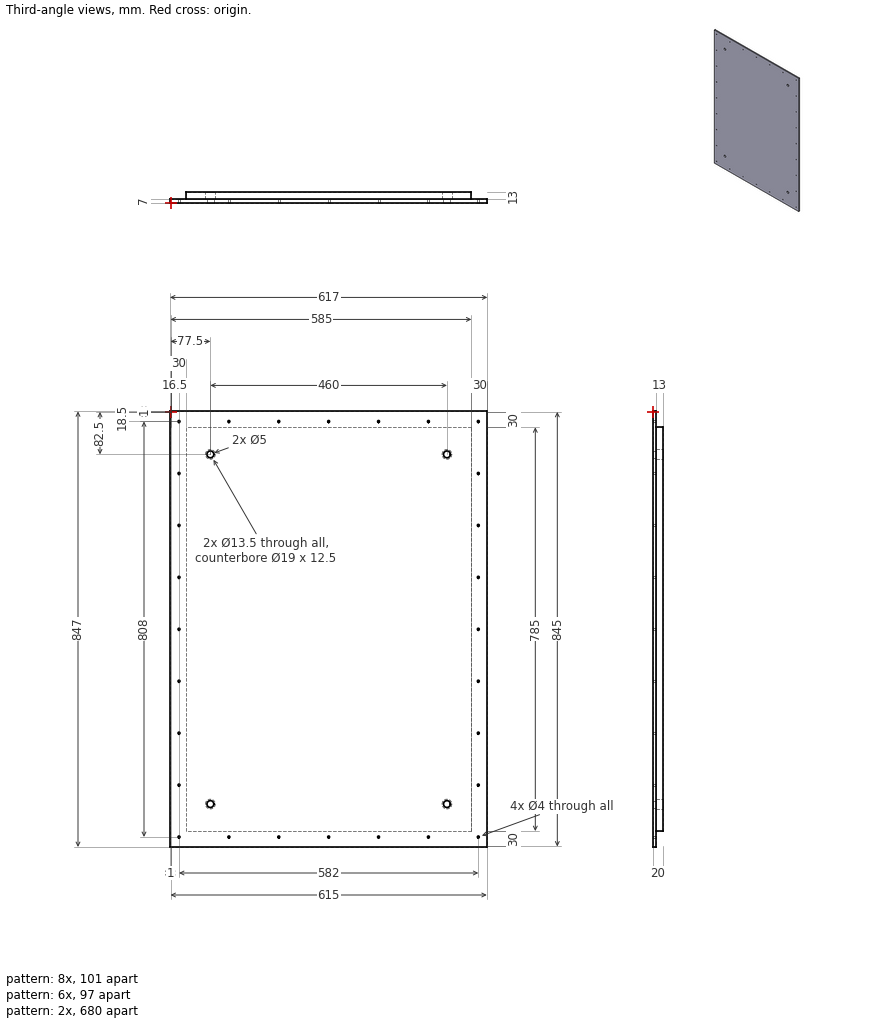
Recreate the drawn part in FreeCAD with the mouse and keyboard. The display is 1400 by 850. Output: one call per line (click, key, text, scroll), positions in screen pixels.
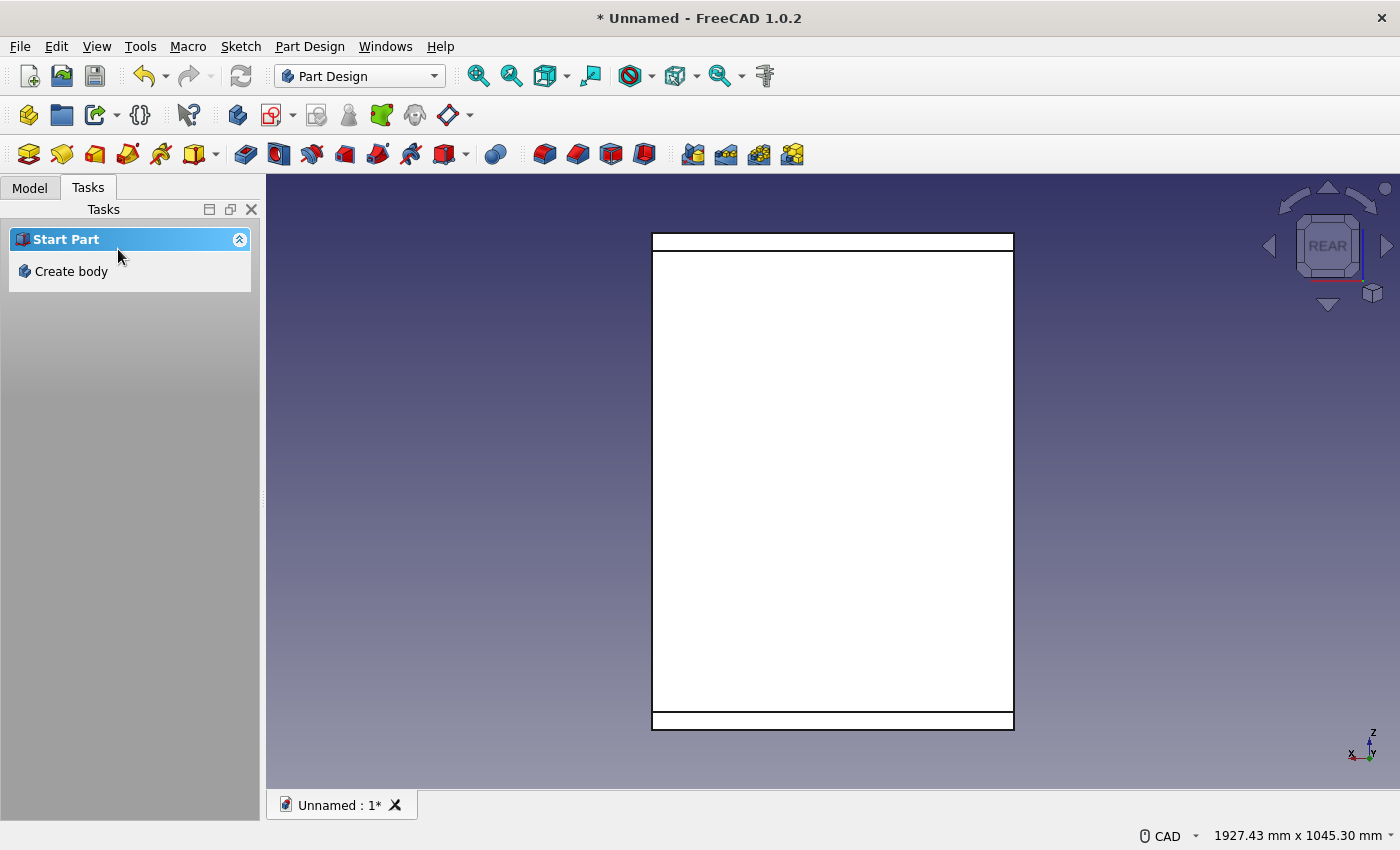
click(833, 480)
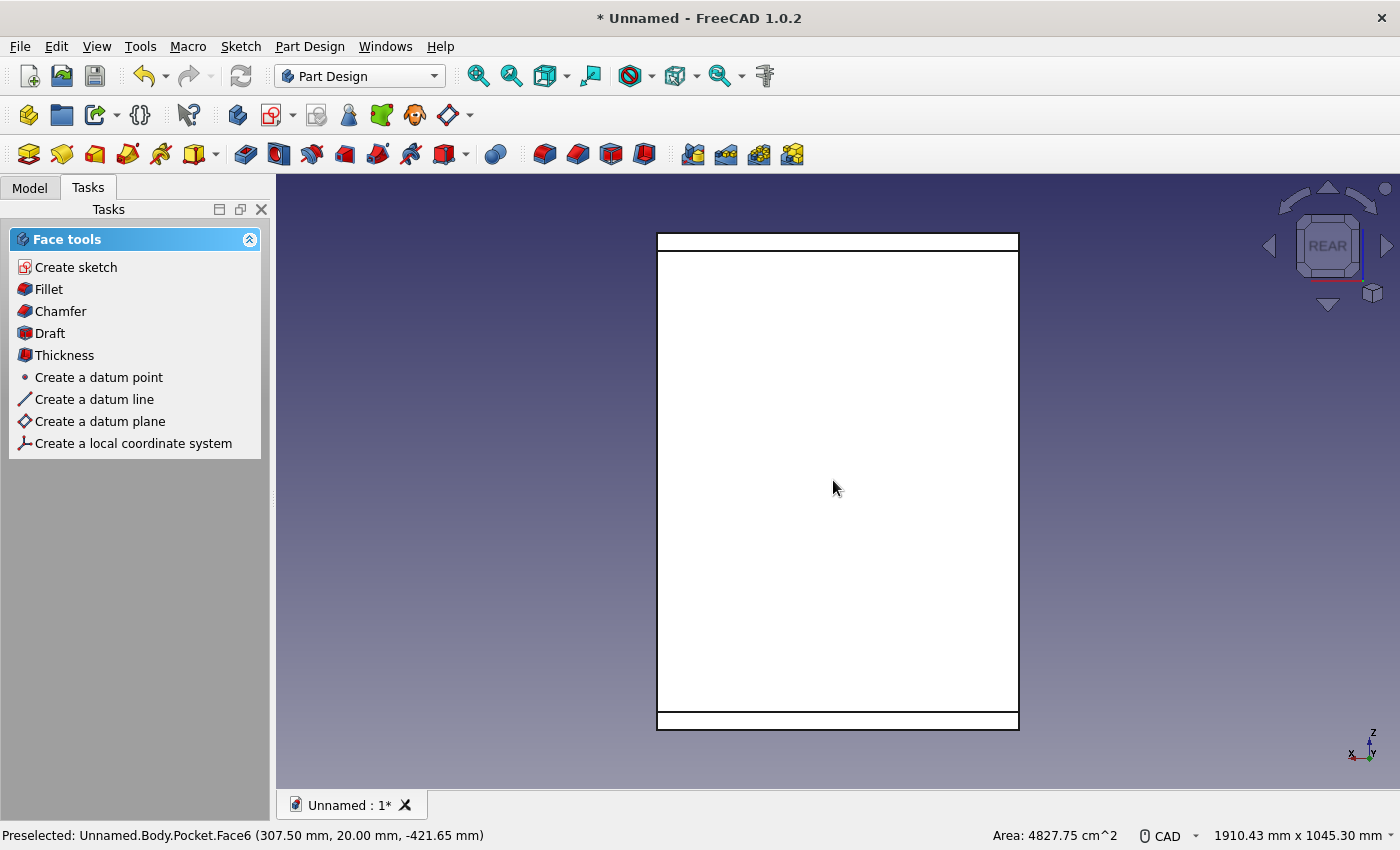
click(270, 116)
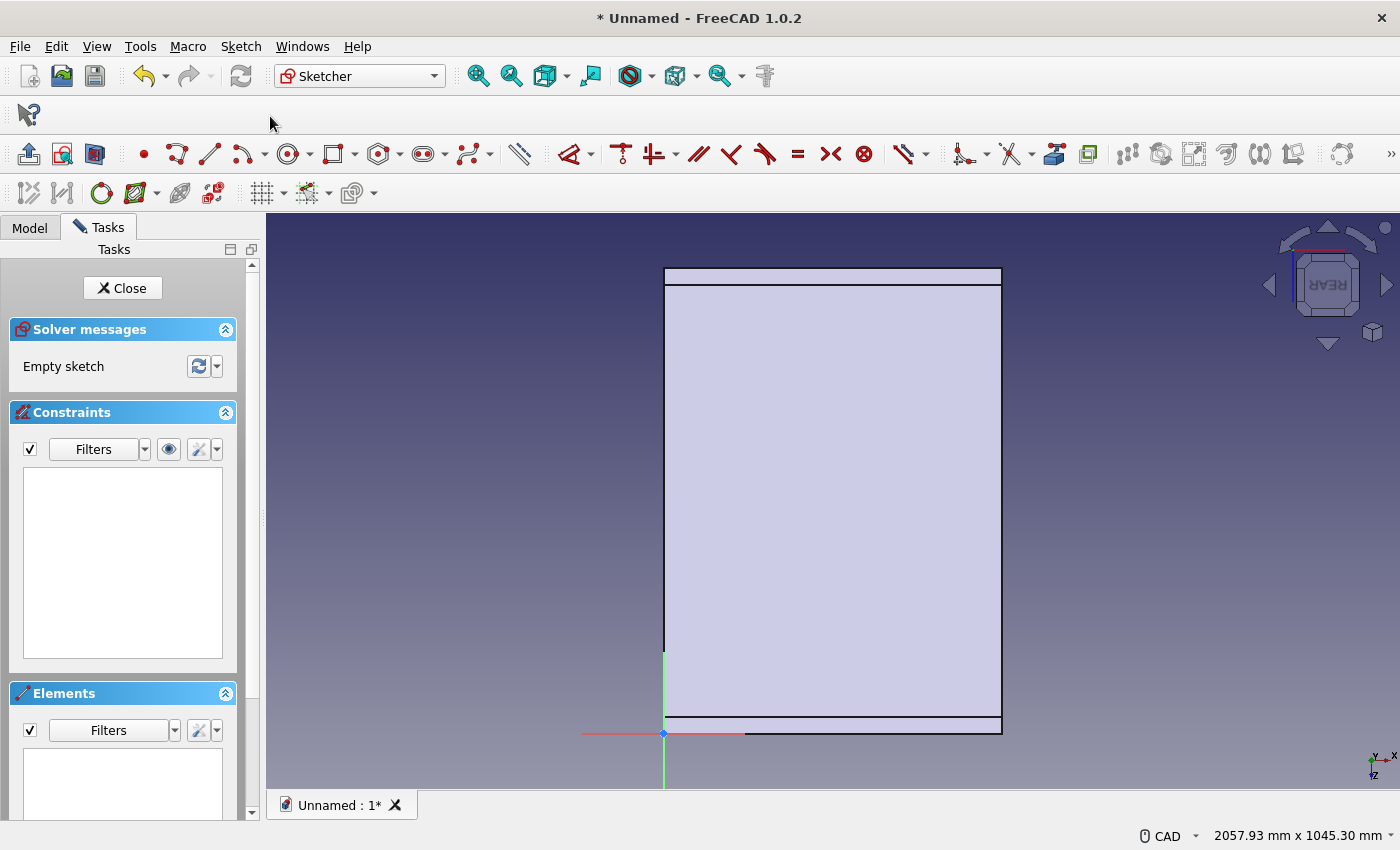
key(g)
key(r)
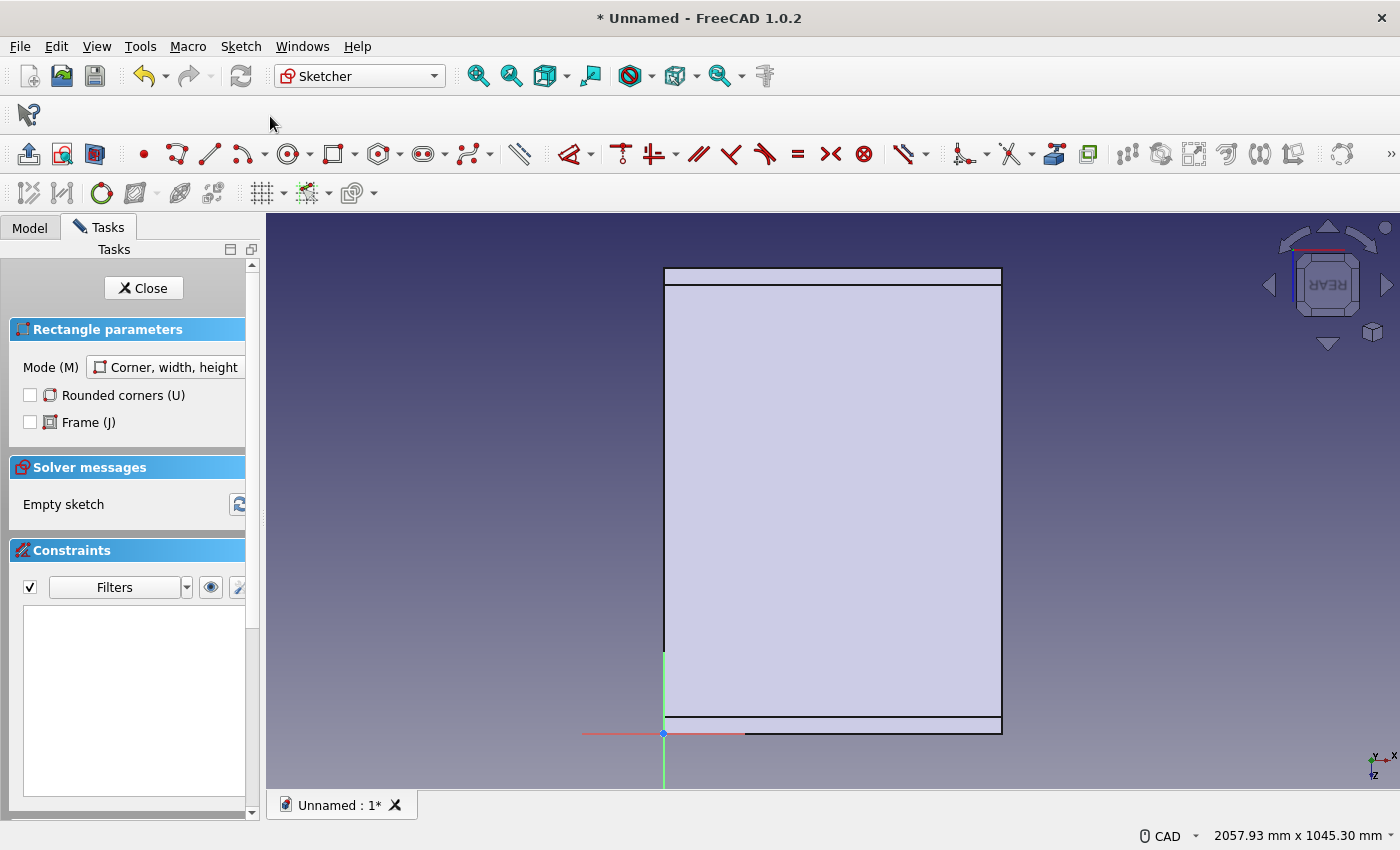
click(986, 285)
move(1002, 717)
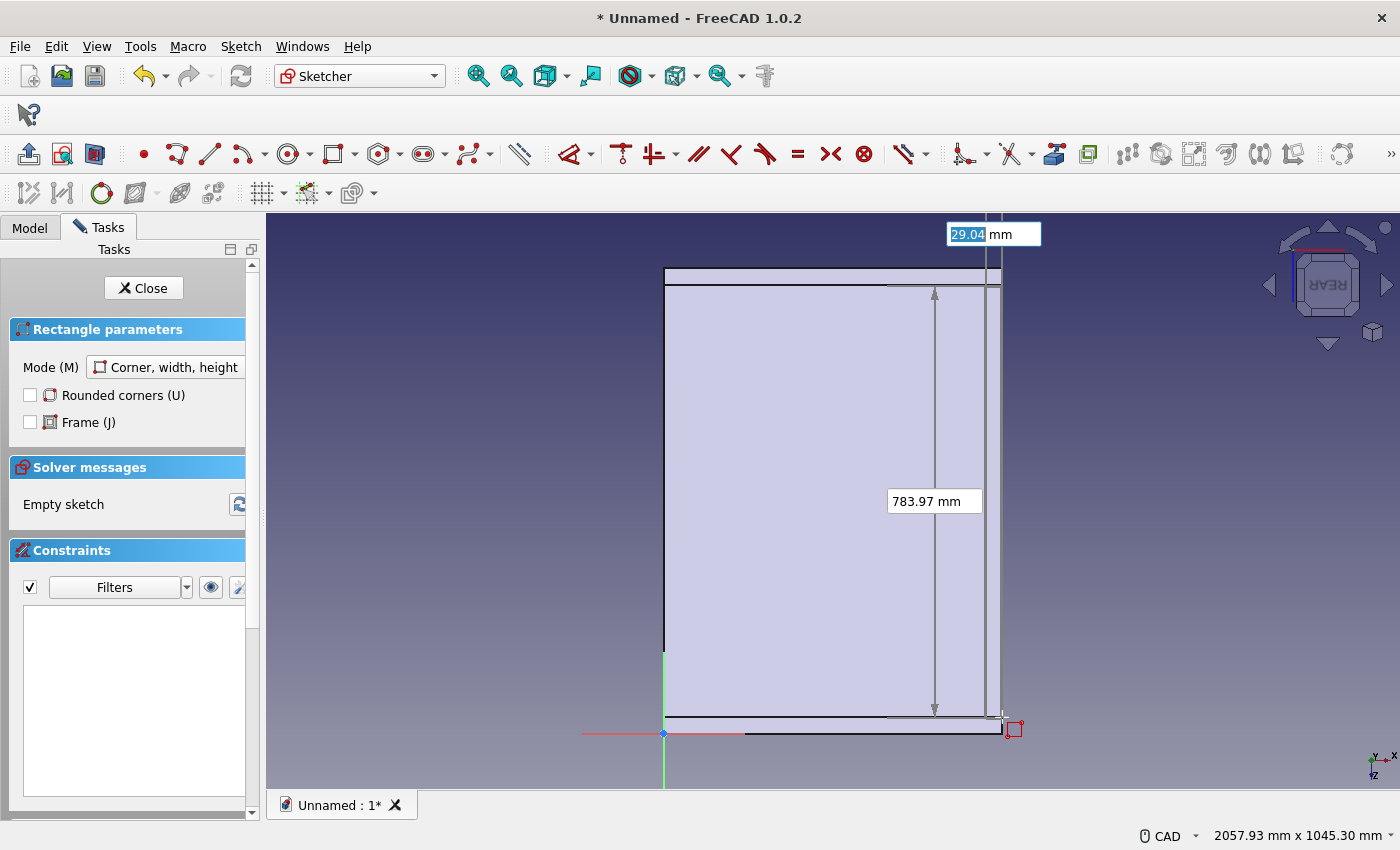
text(30)
key(Tab)
text(785)
key(Return)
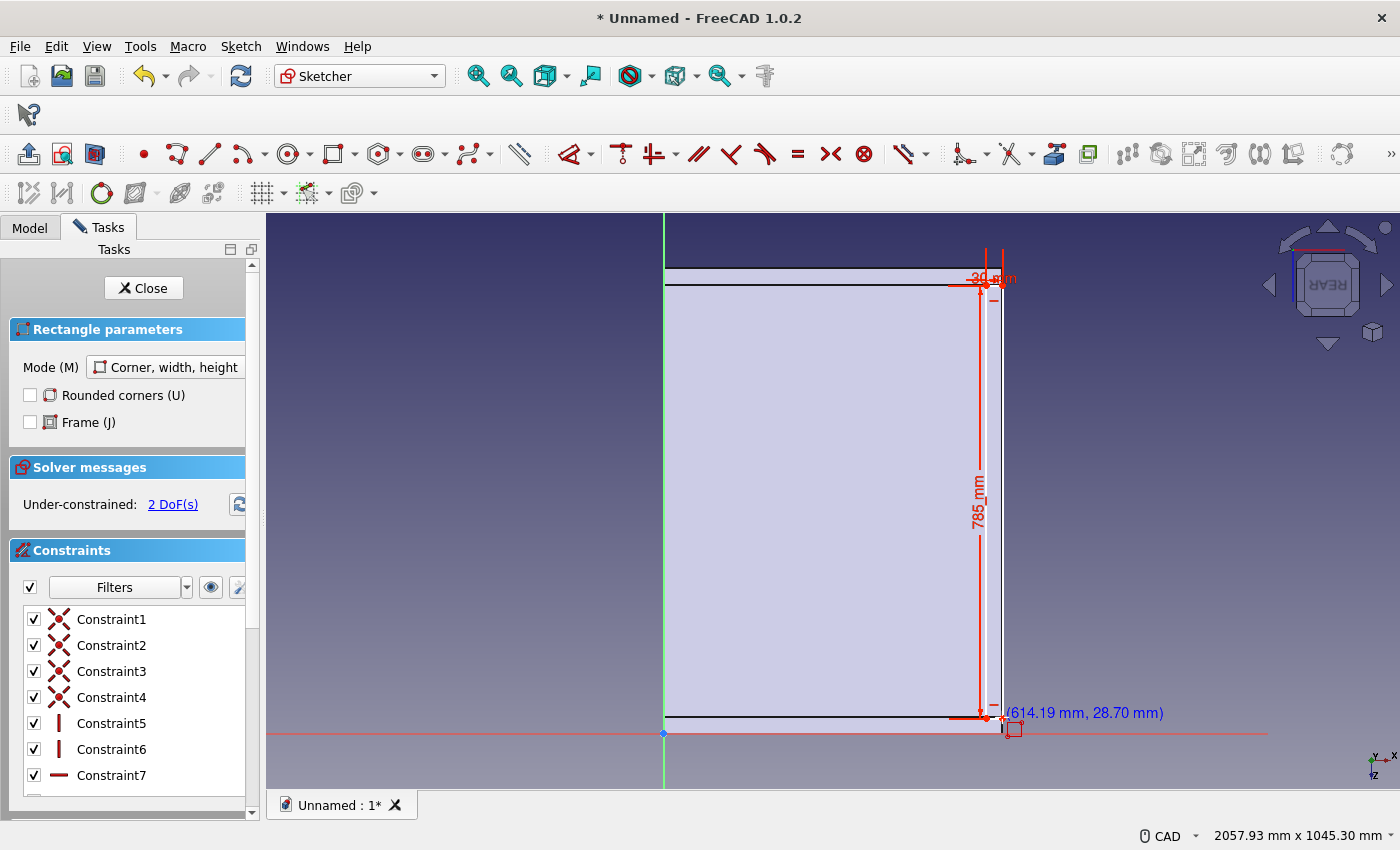
click(664, 285)
move(680, 717)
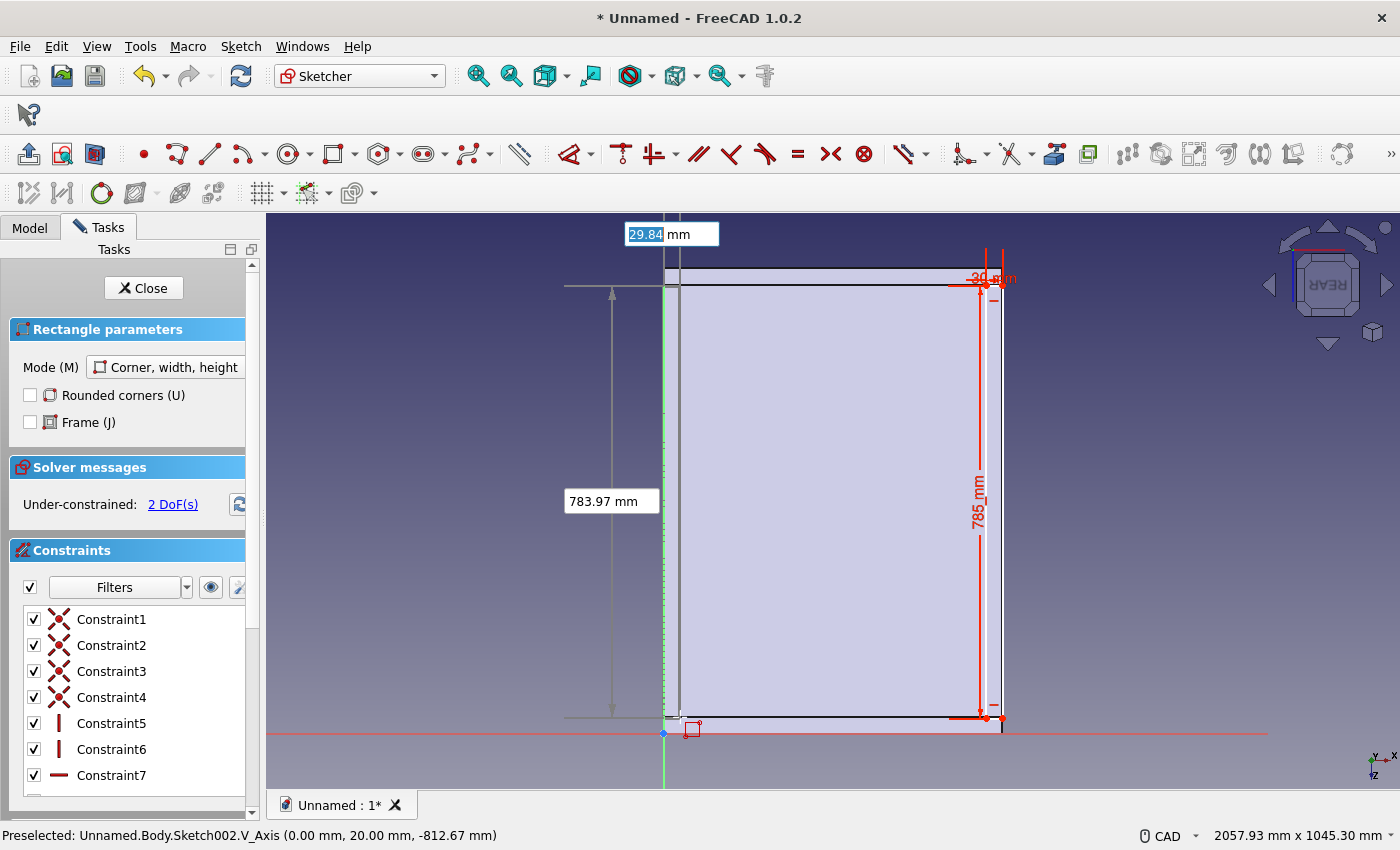
text(30)
key(Tab)
text(785)
key(Return)
key(Escape)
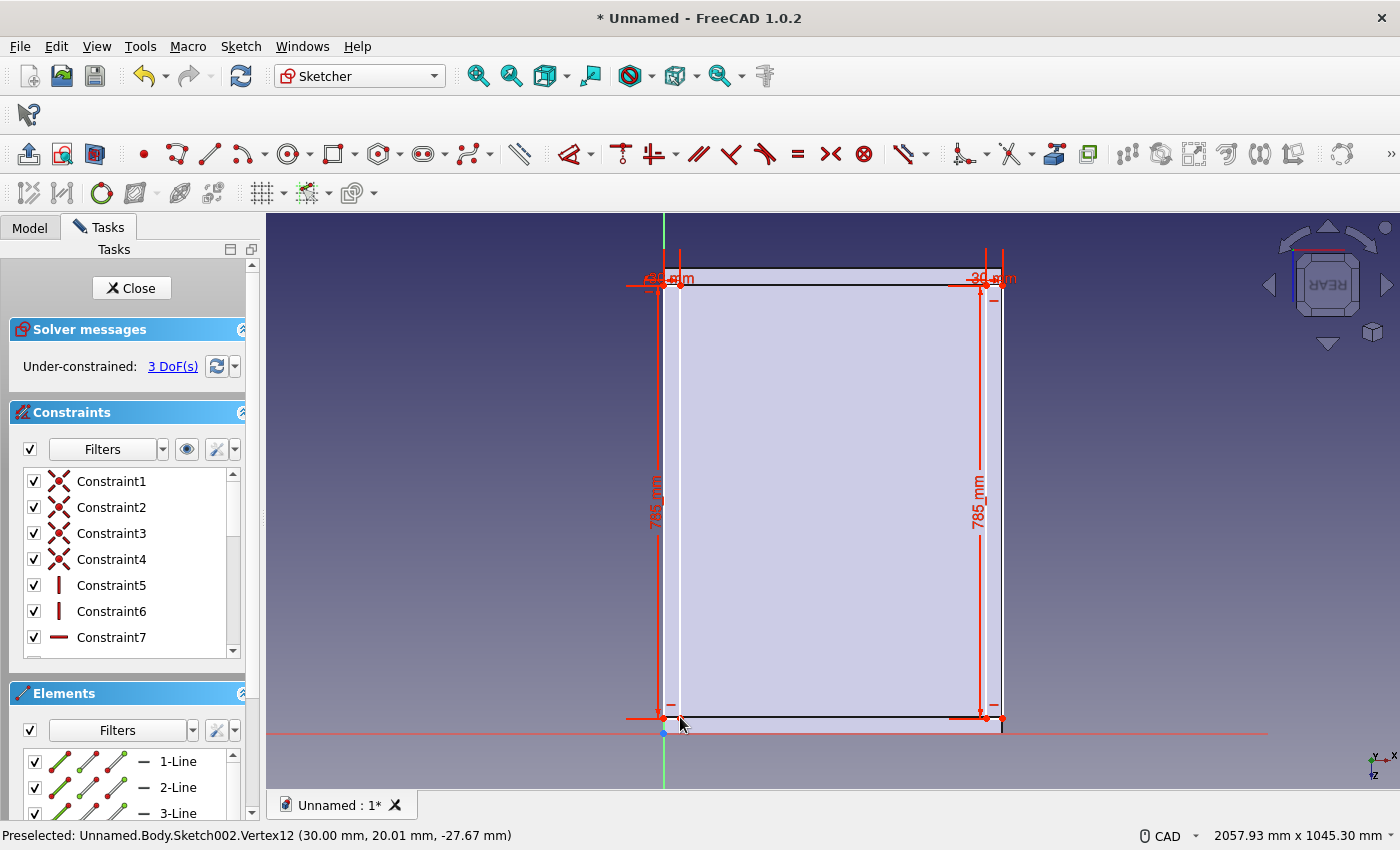
key(d)